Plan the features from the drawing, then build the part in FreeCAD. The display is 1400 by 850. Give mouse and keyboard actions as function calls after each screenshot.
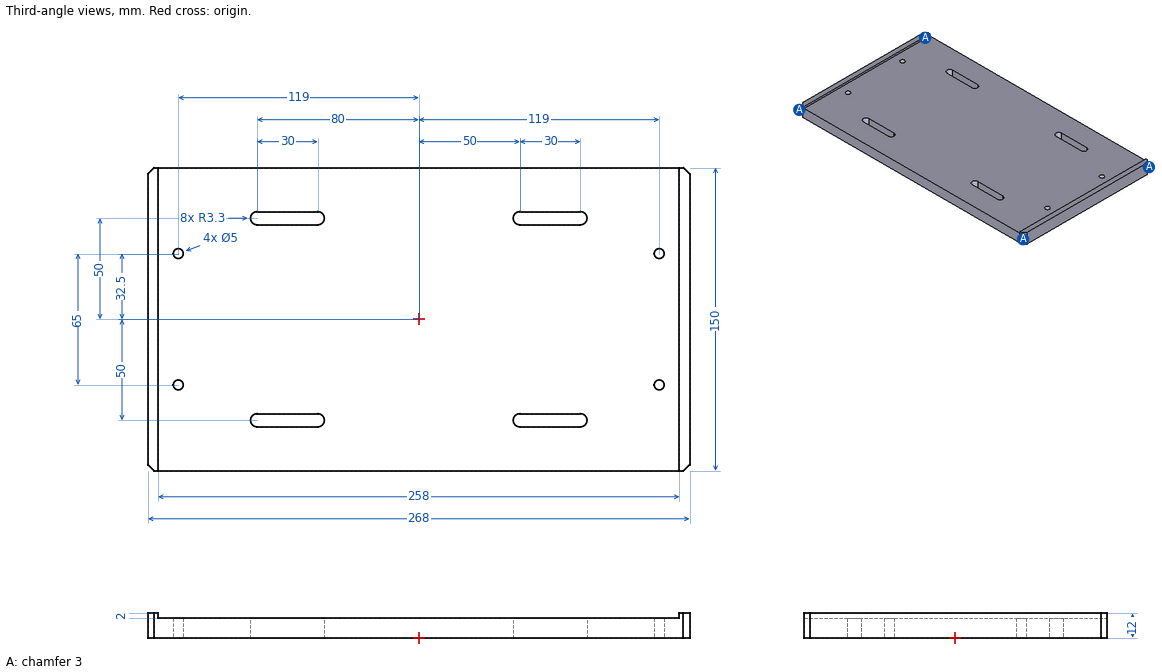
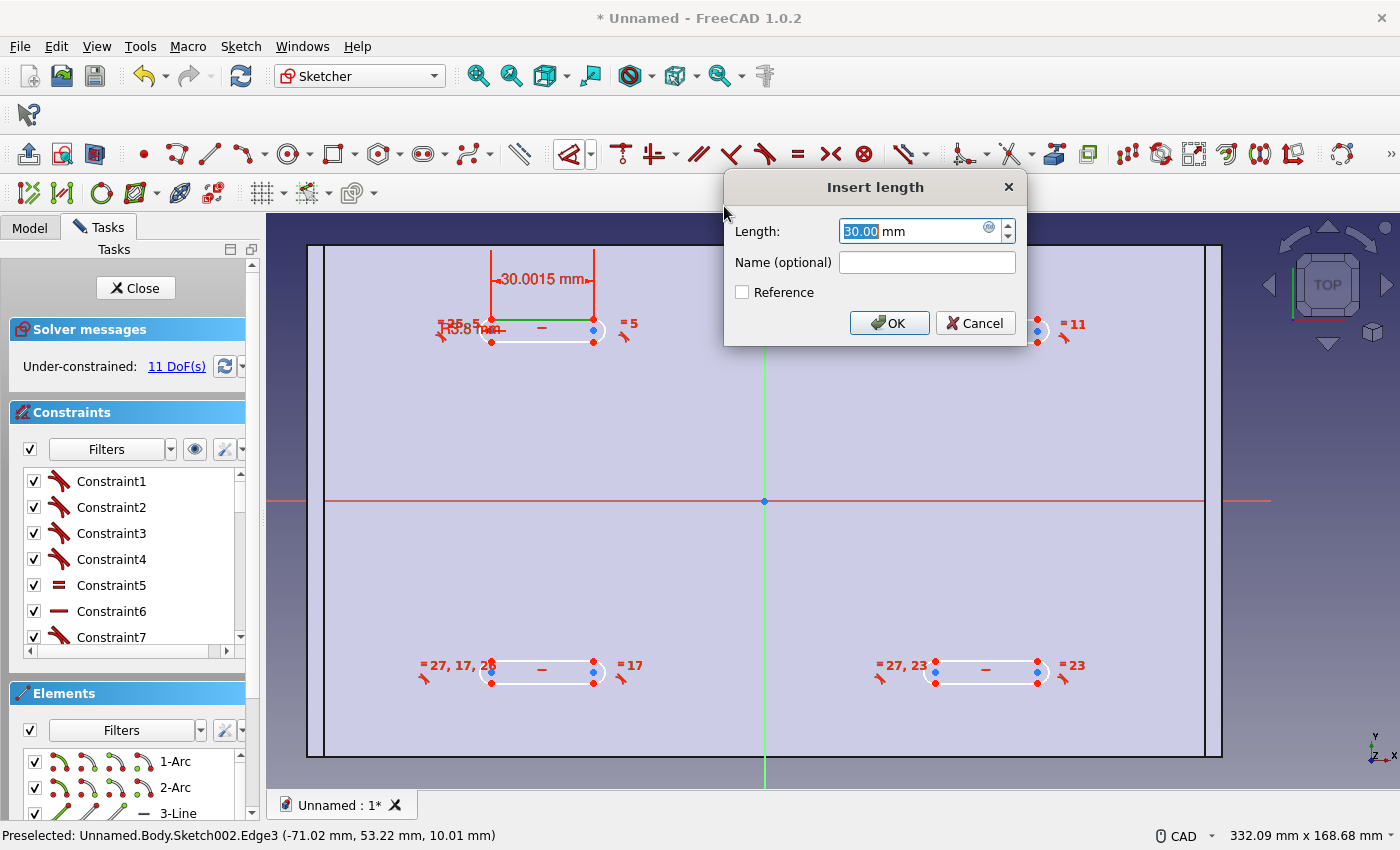
text(30)
key(Return)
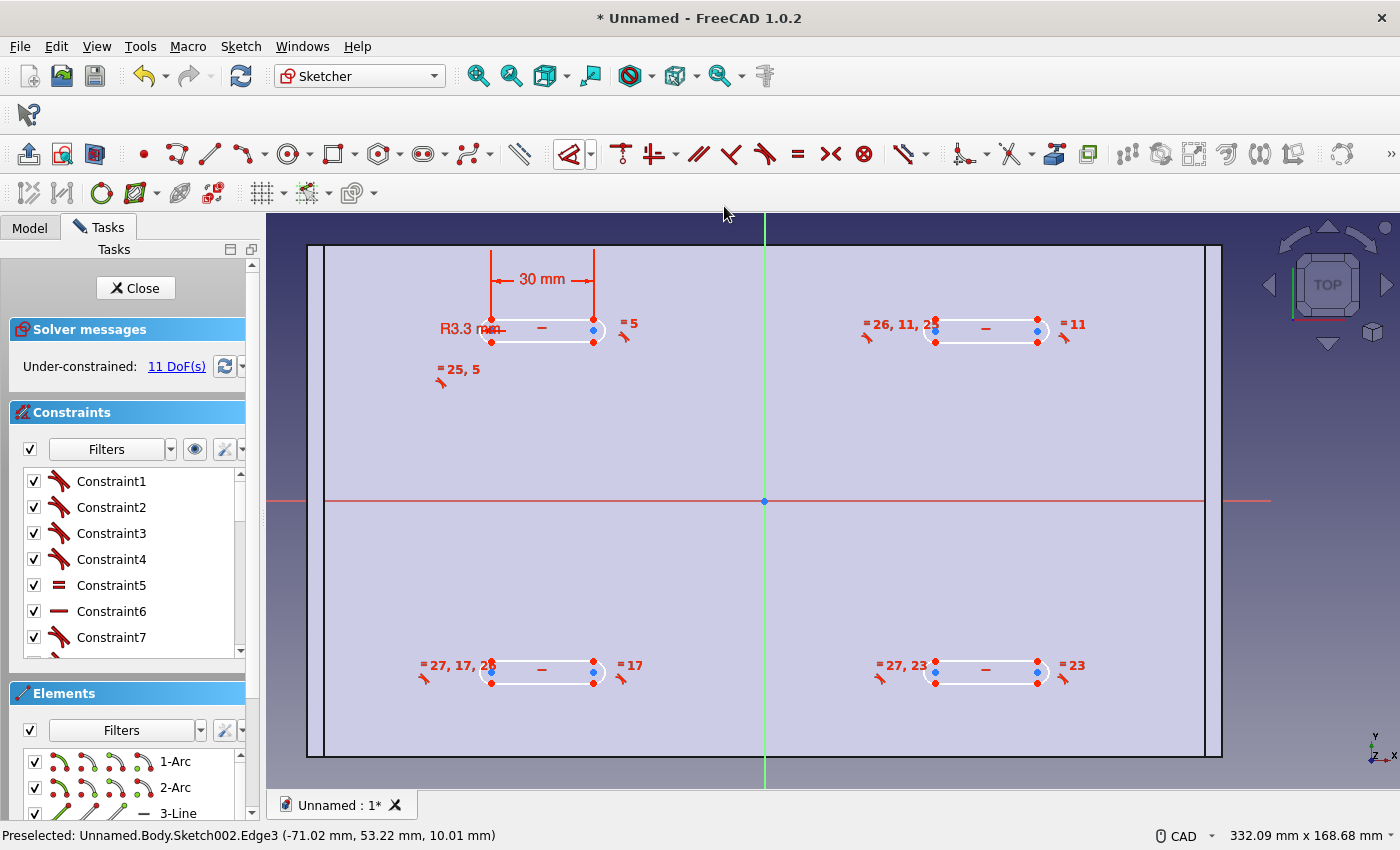
click(966, 320)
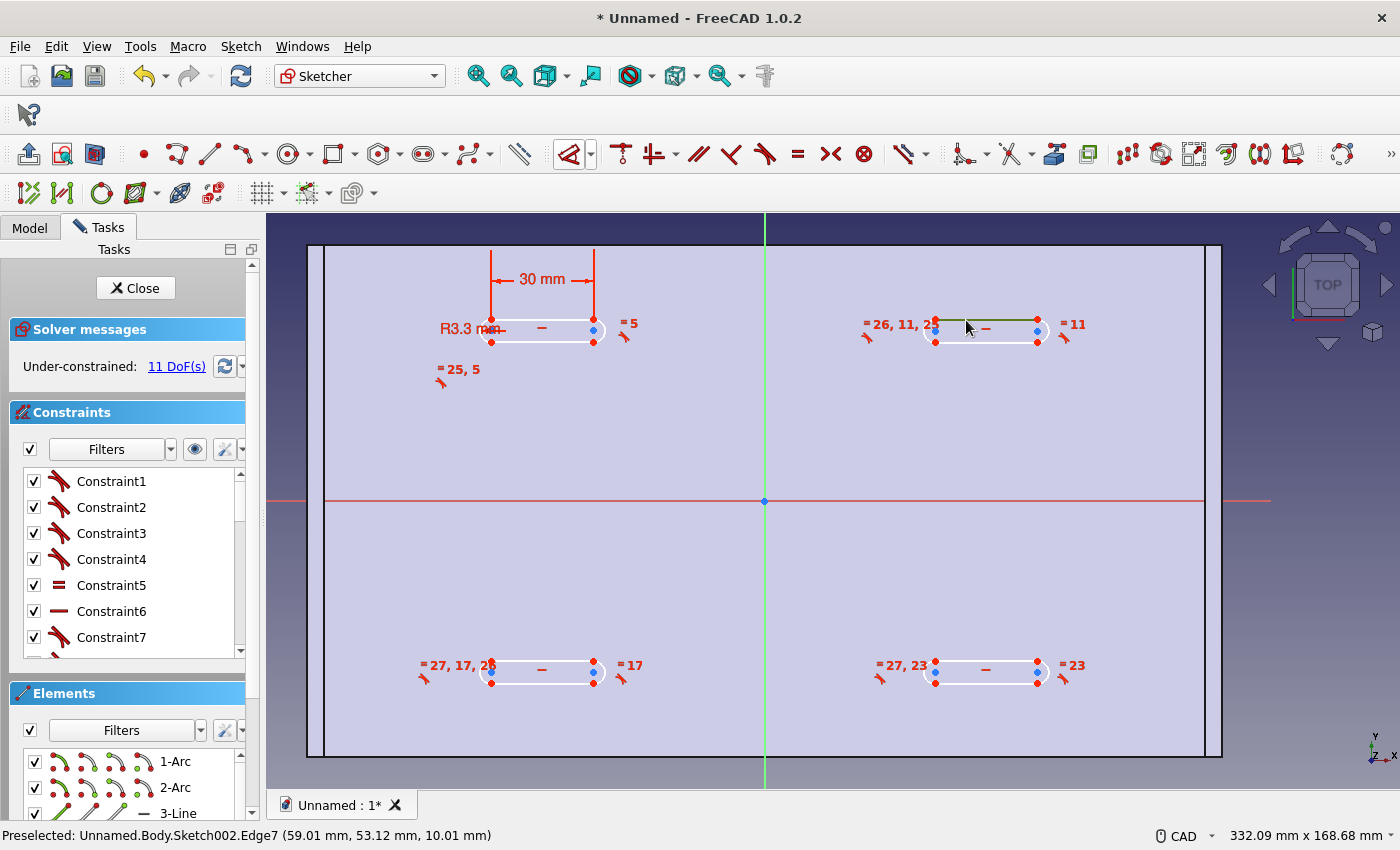
key(l)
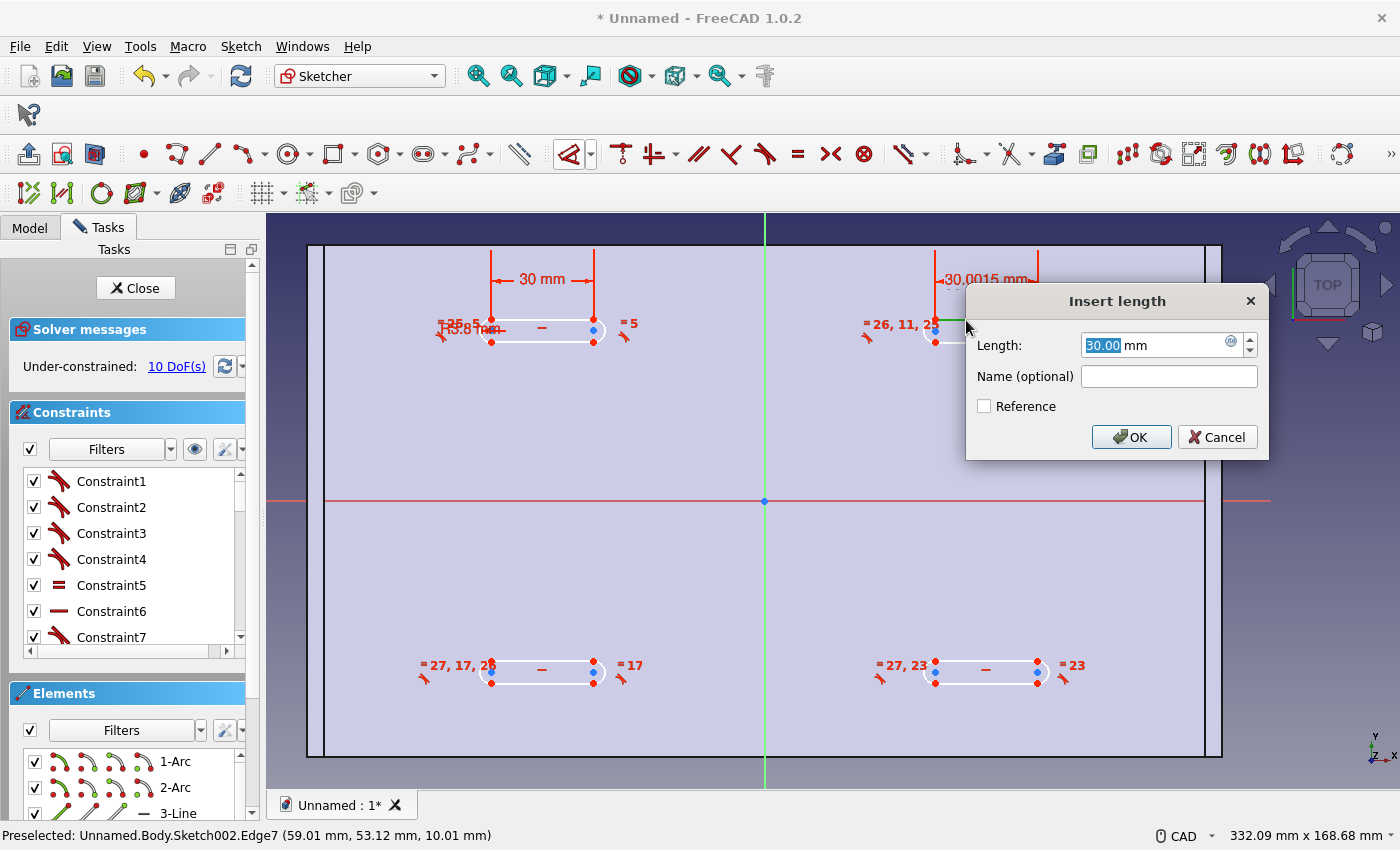
text(30)
key(Return)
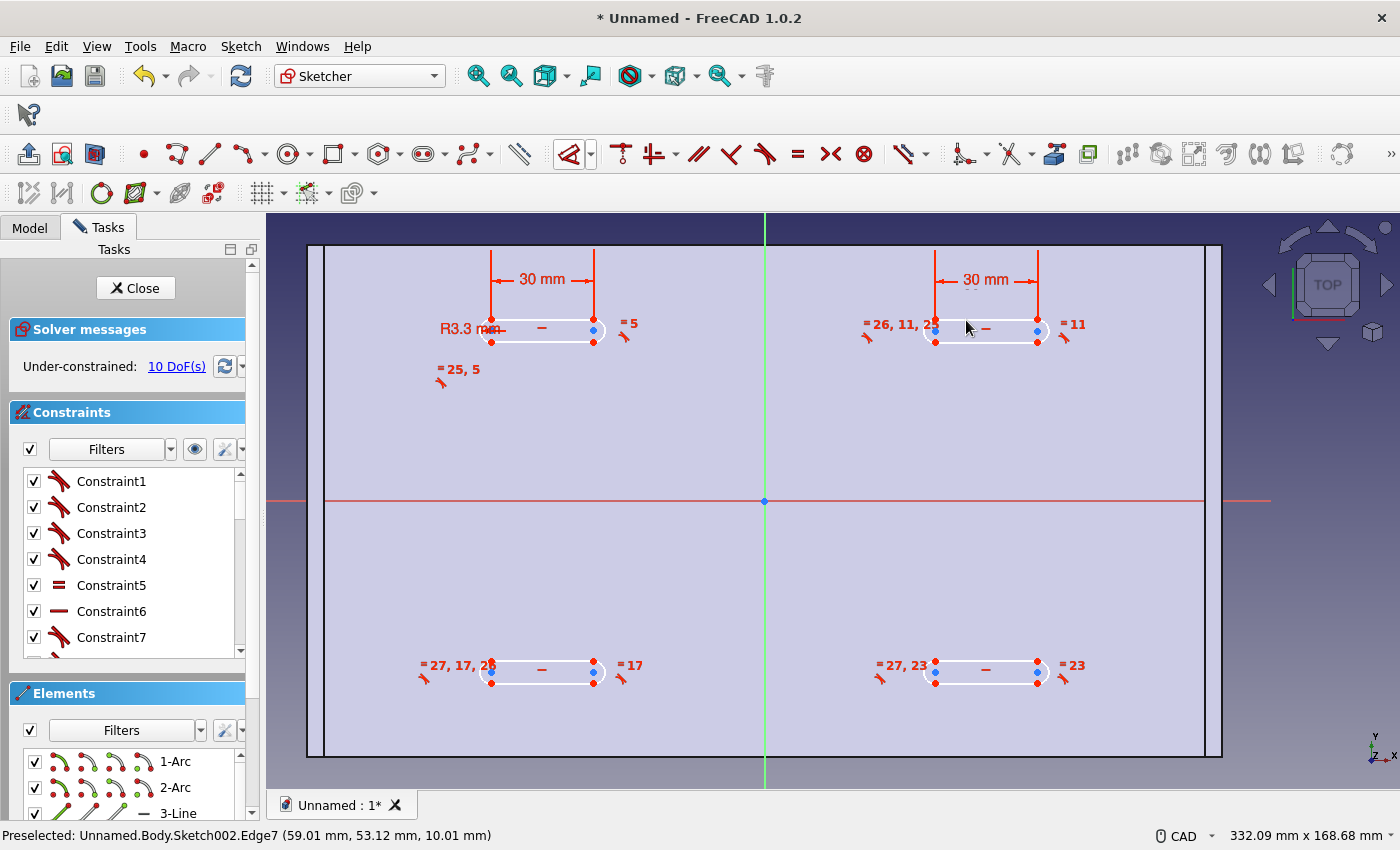
click(522, 661)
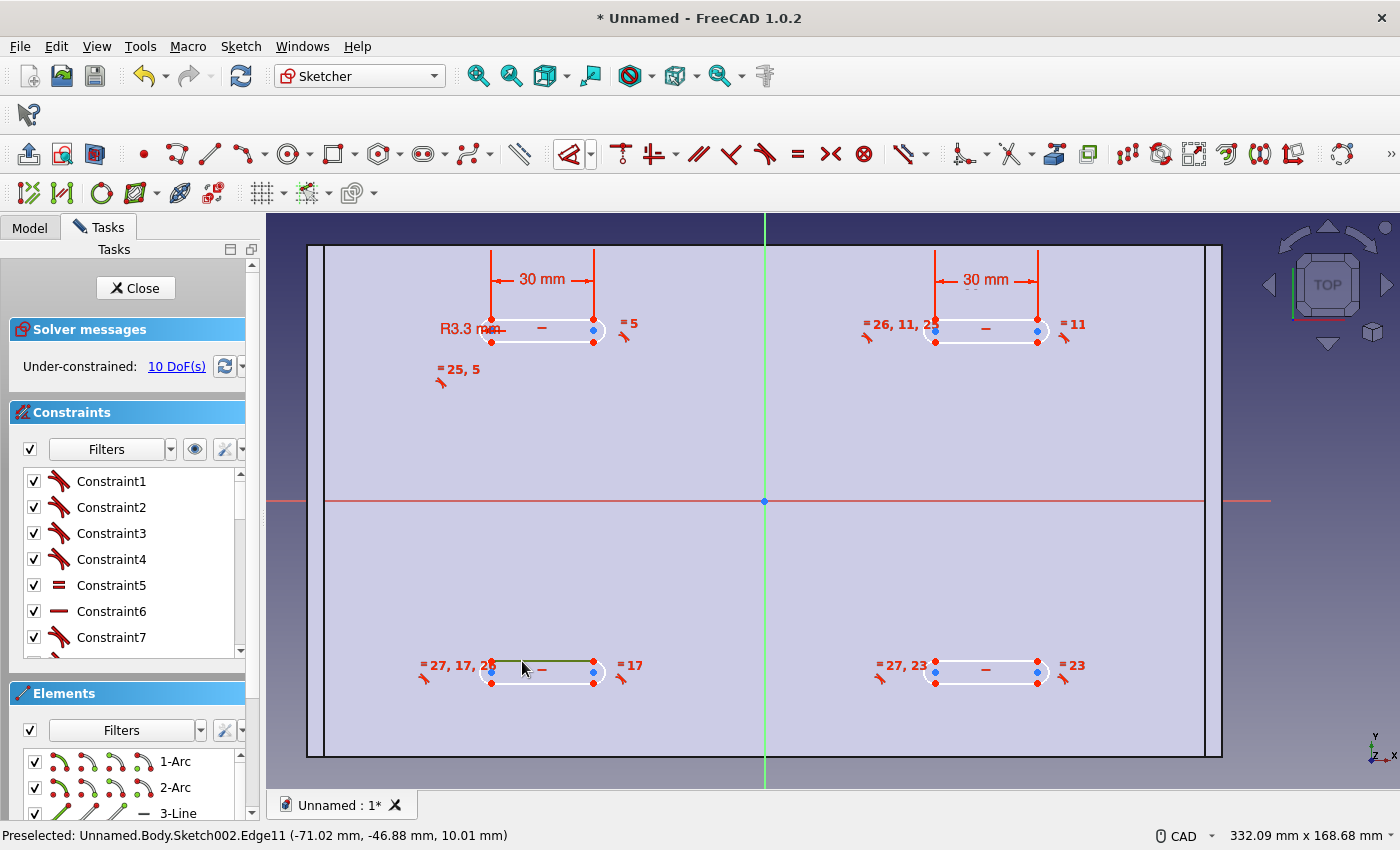
click(590, 154)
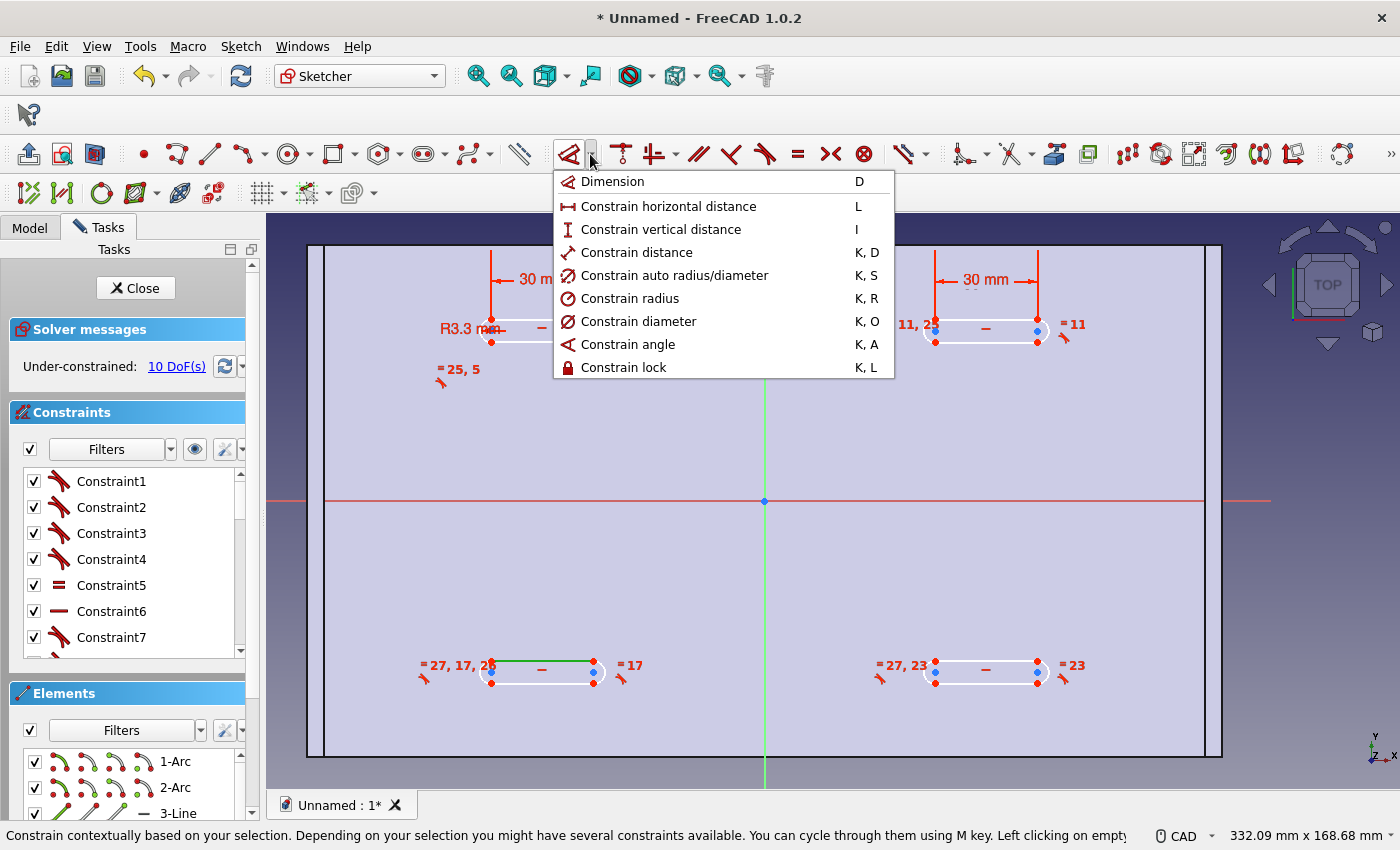
click(724, 206)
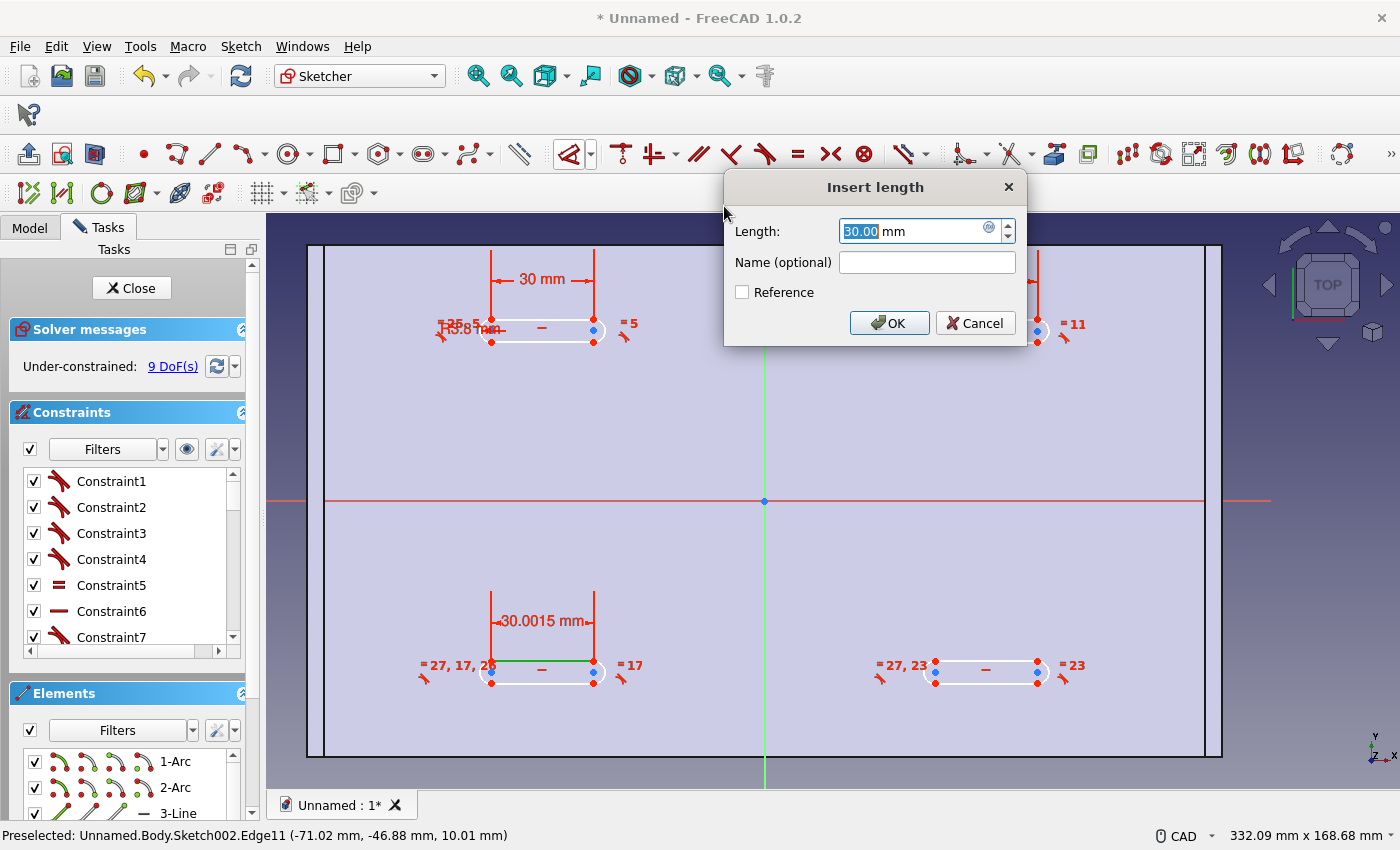
text(30)
key(Return)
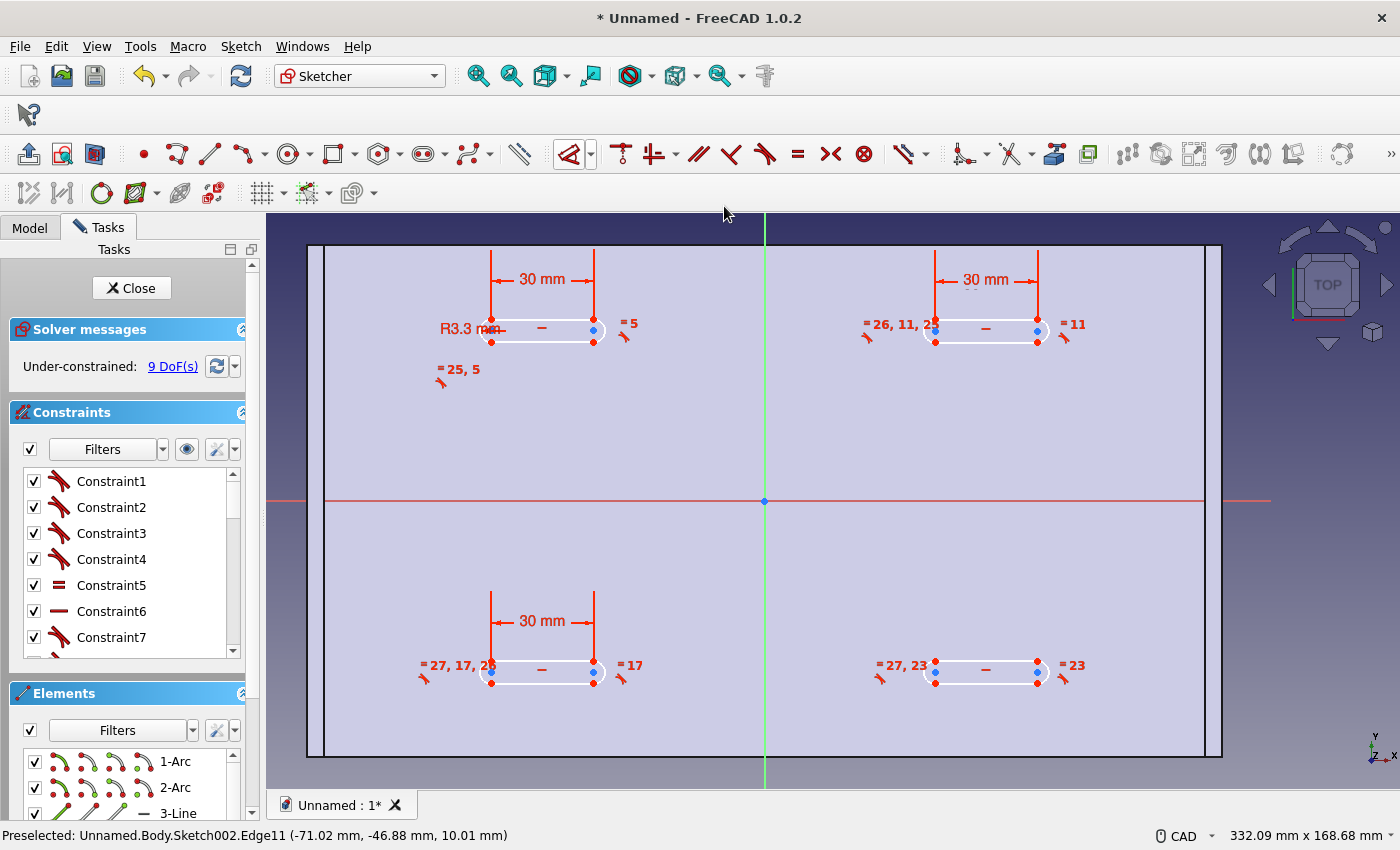
click(966, 661)